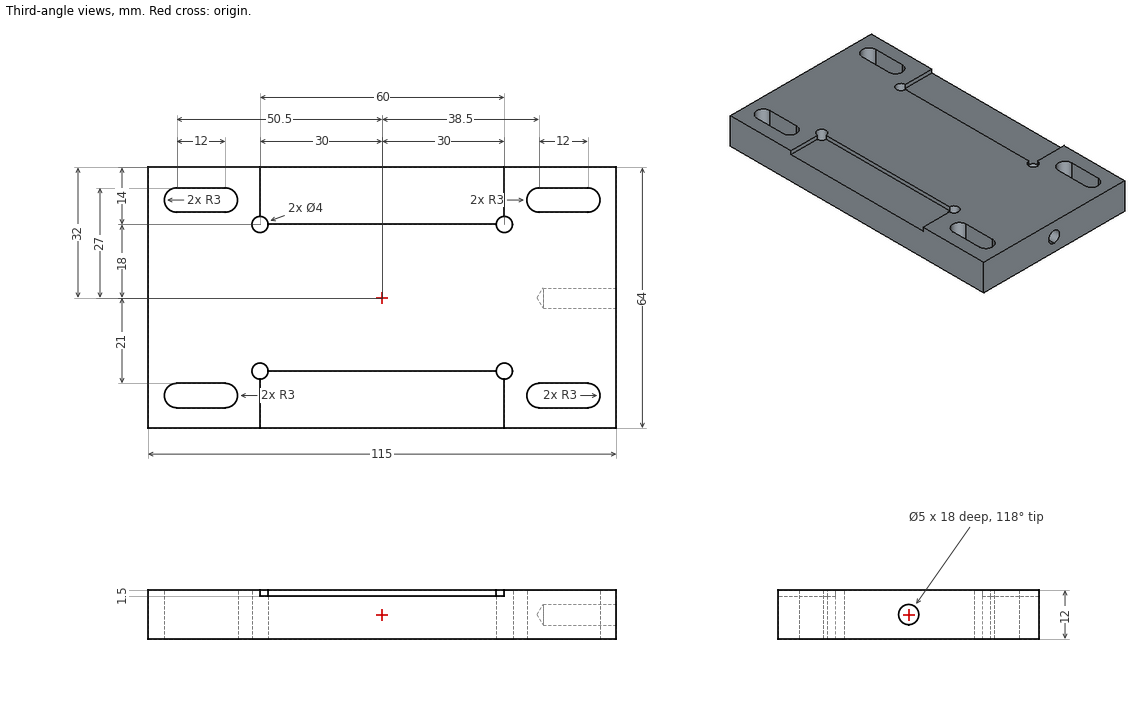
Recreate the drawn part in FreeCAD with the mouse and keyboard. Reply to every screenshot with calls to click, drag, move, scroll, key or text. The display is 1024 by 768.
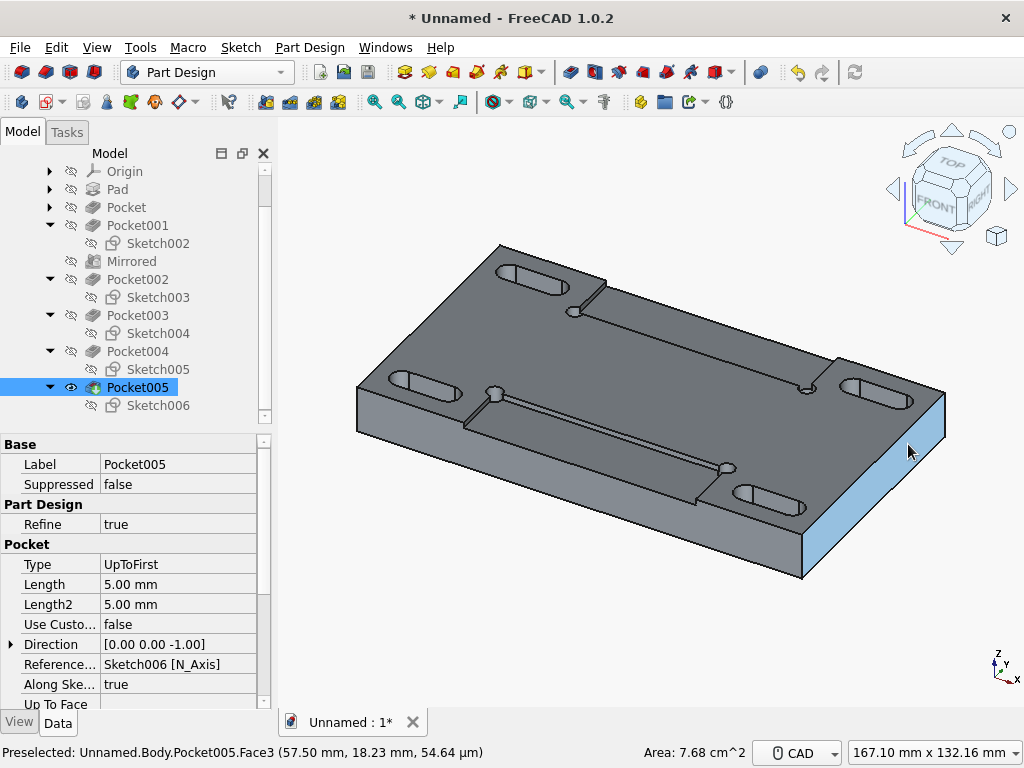
click(46, 102)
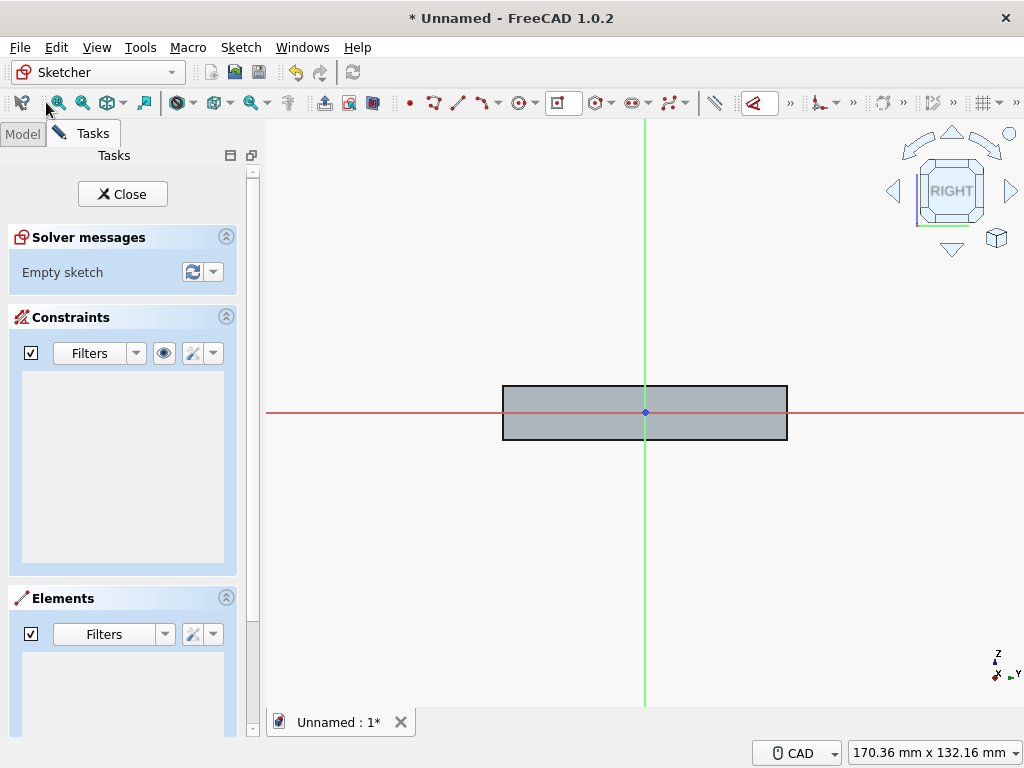
scroll(649, 413, up, 14)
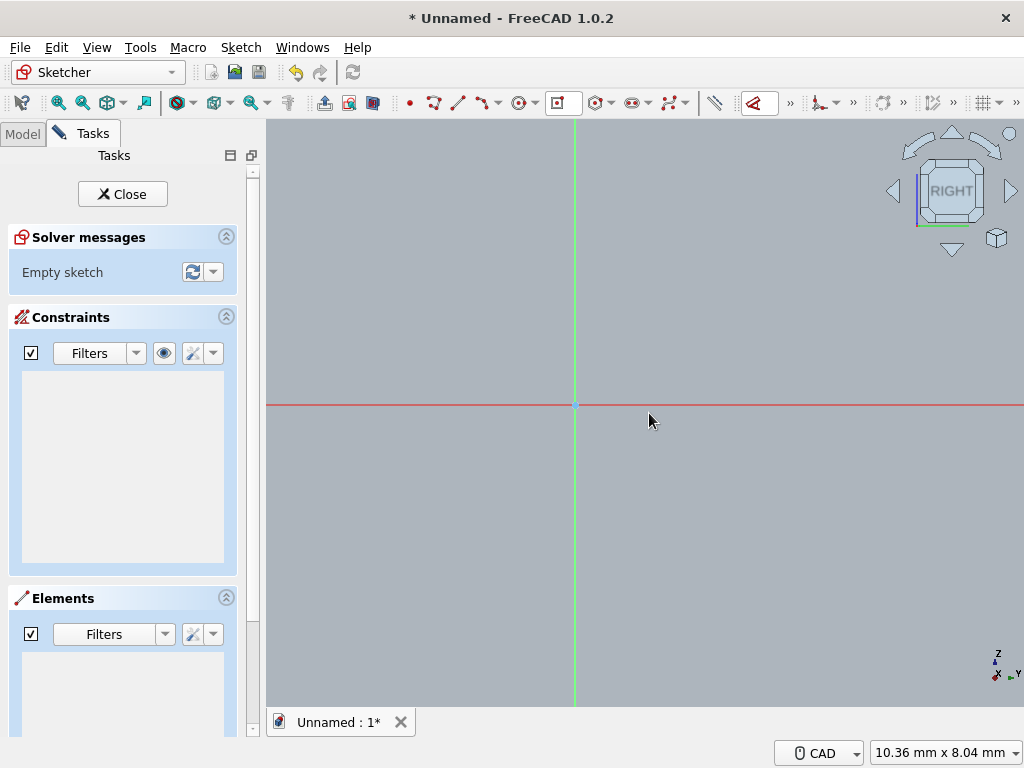
click(520, 104)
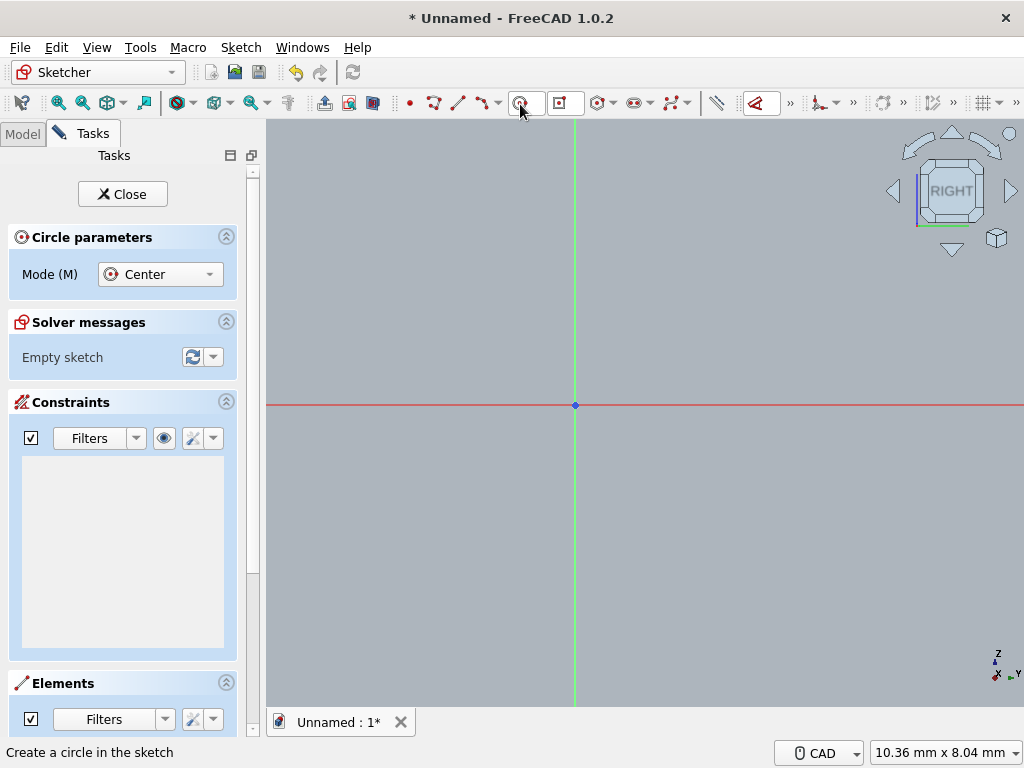
click(575, 405)
click(705, 276)
key(Escape)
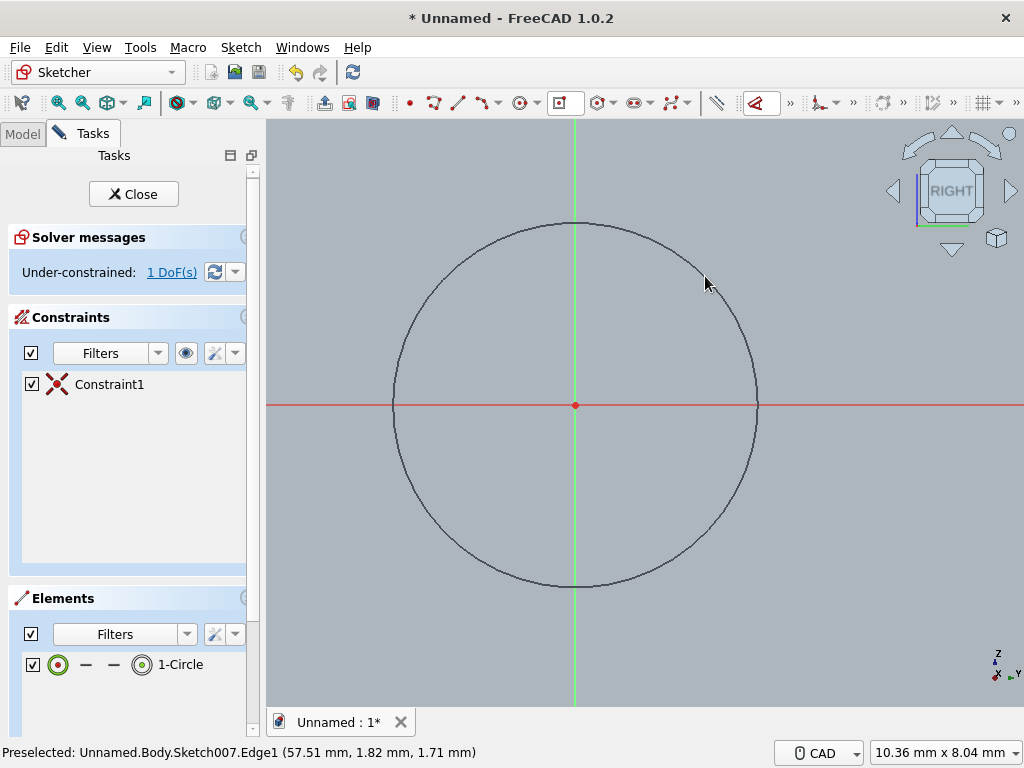
click(704, 276)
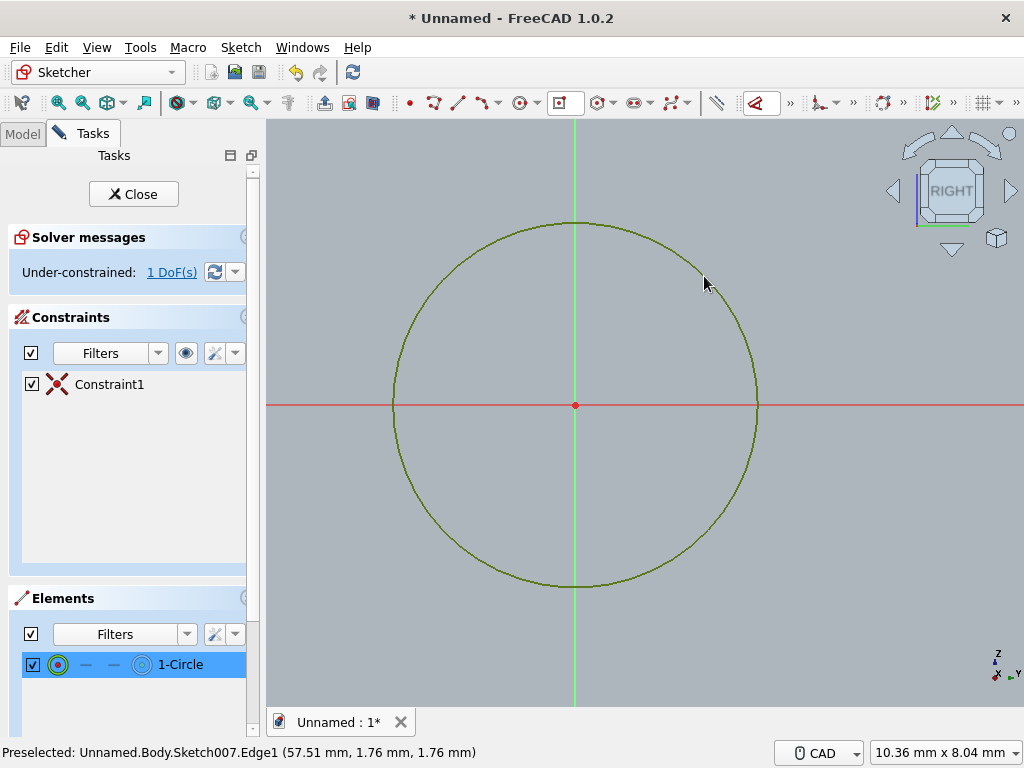
click(774, 104)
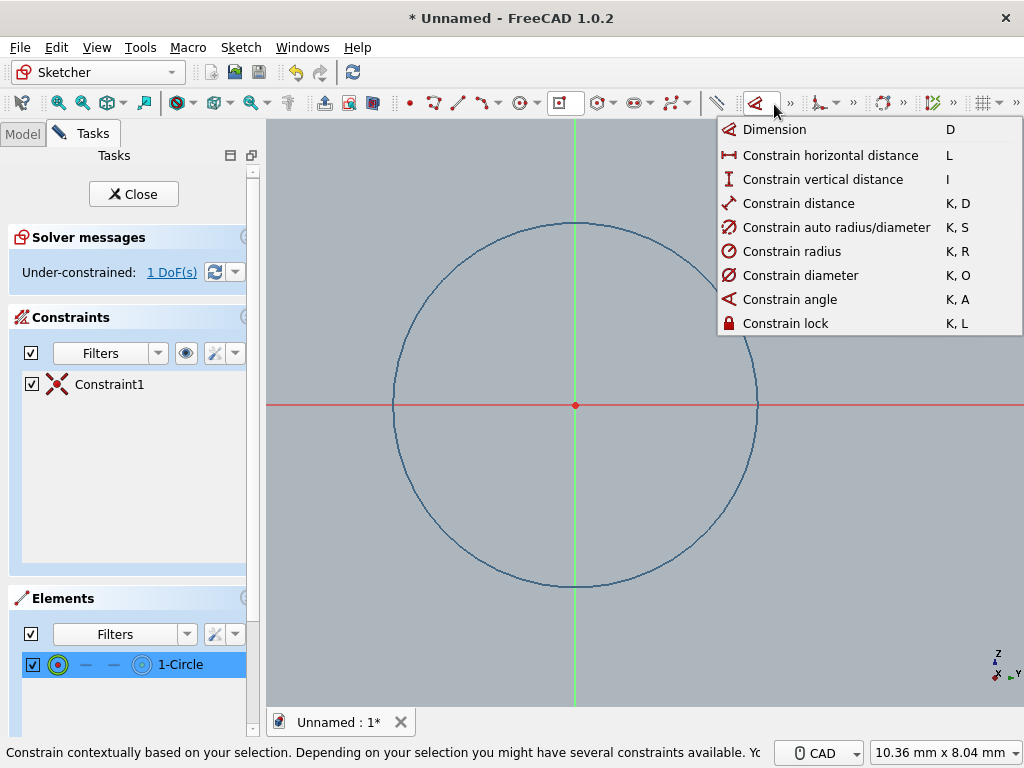
click(870, 275)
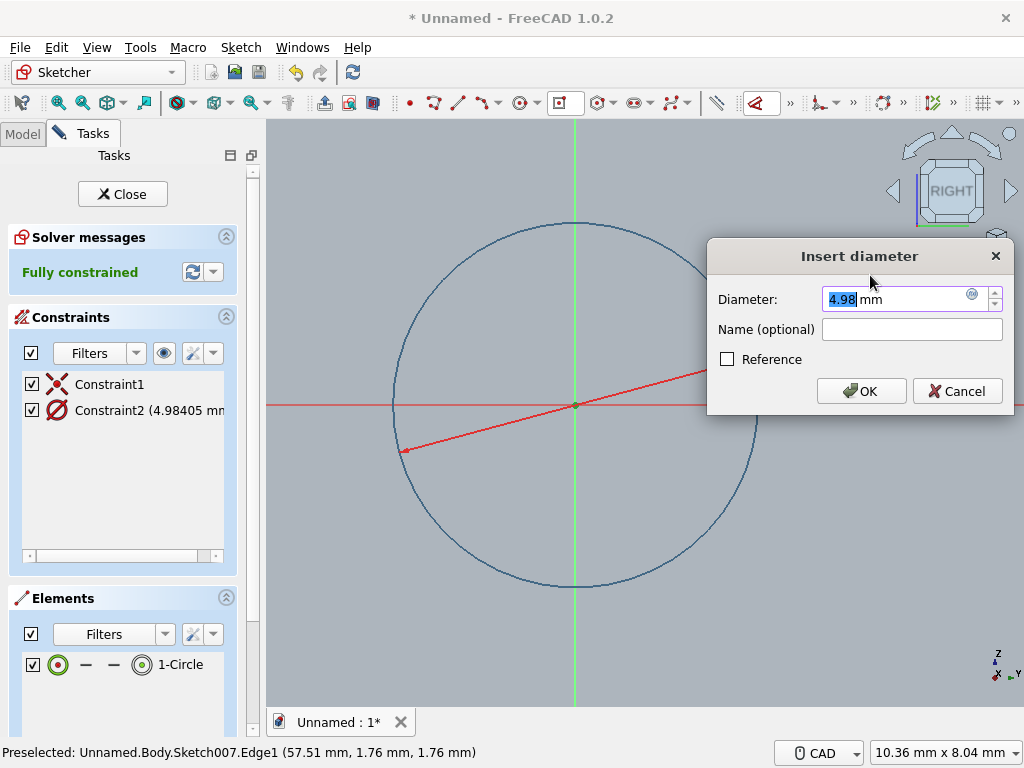
text(5)
key(Return)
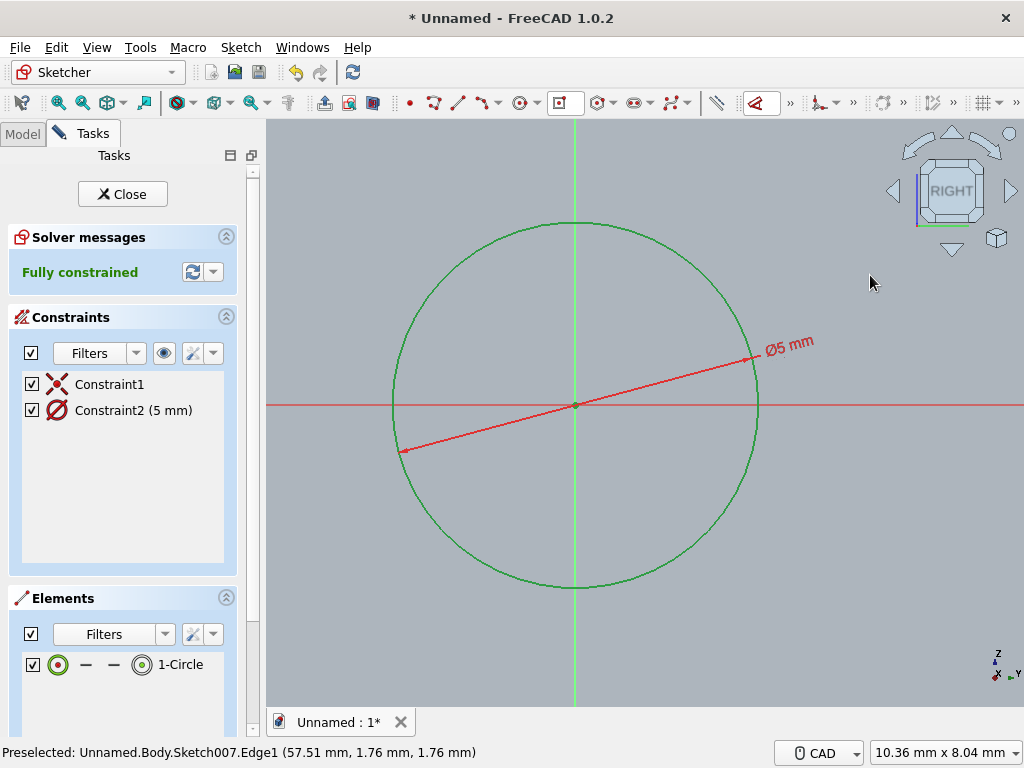
click(123, 194)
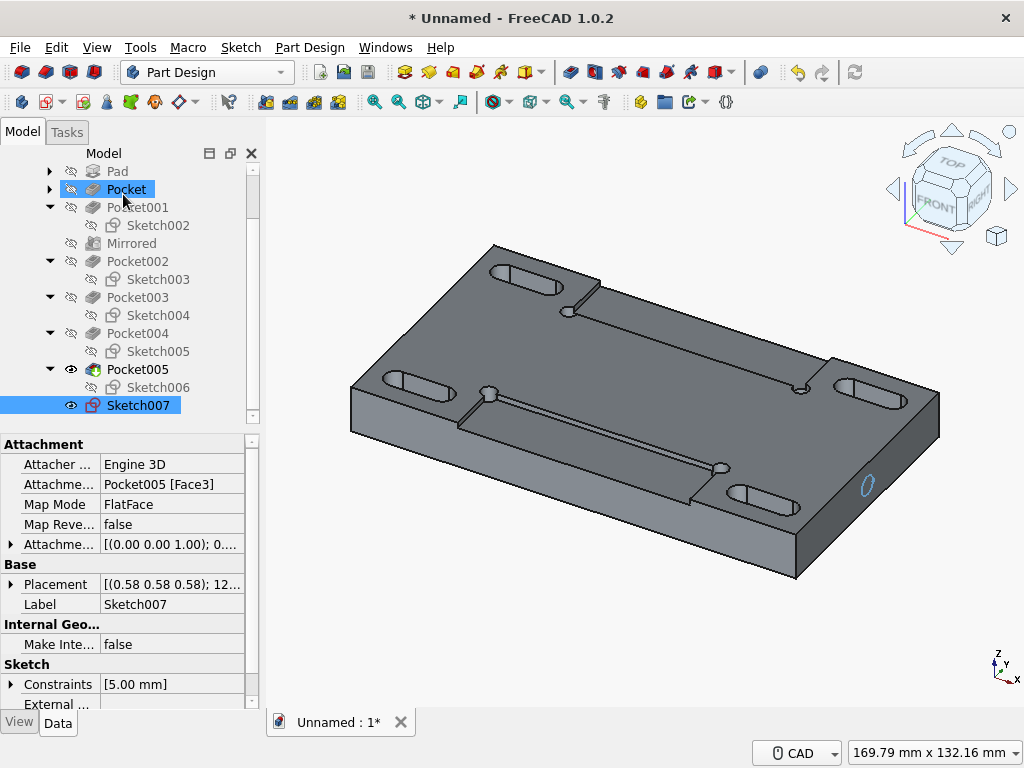
click(596, 72)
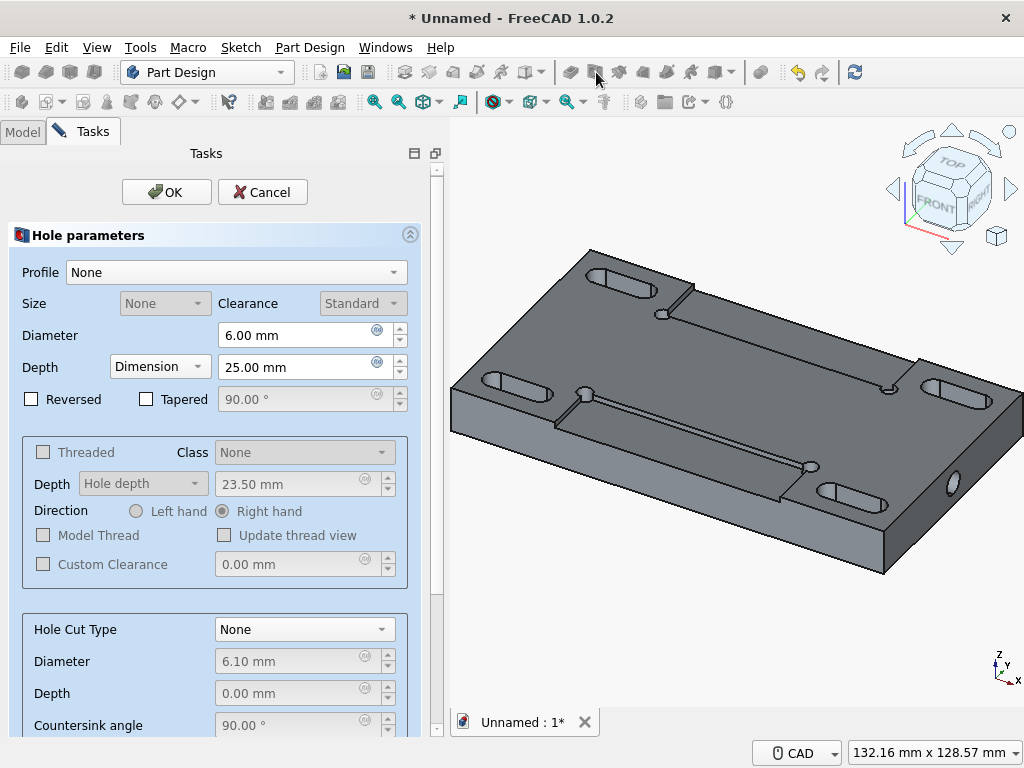
triple_click(305, 335)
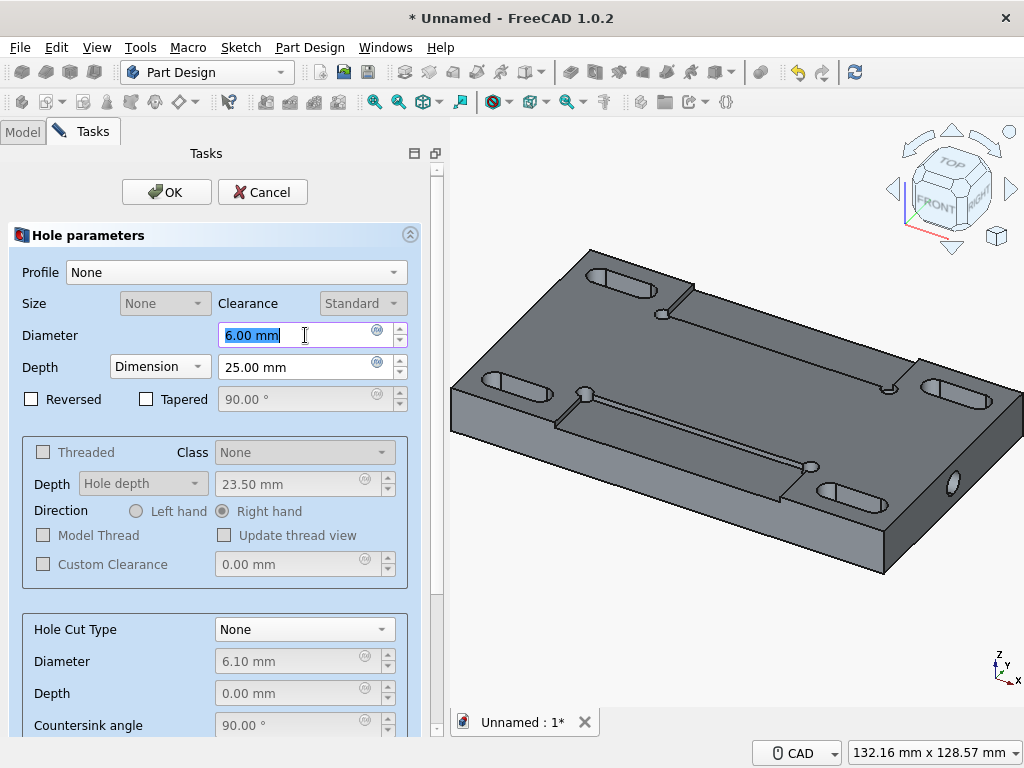
text(5)
key(Tab)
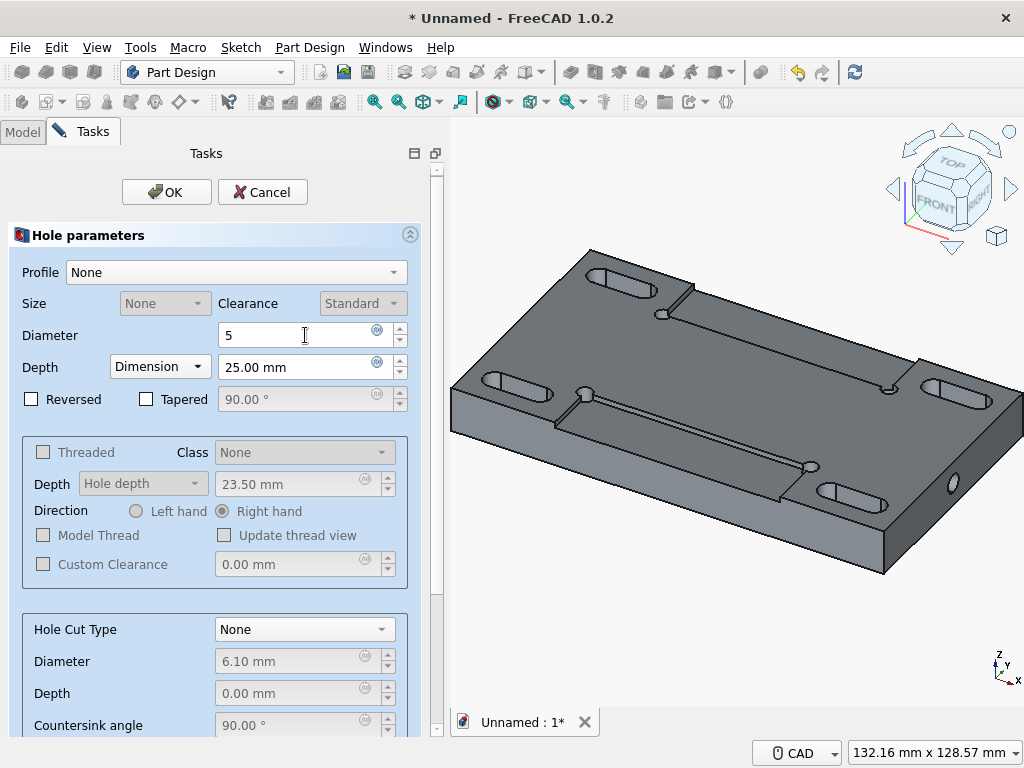
triple_click(305, 367)